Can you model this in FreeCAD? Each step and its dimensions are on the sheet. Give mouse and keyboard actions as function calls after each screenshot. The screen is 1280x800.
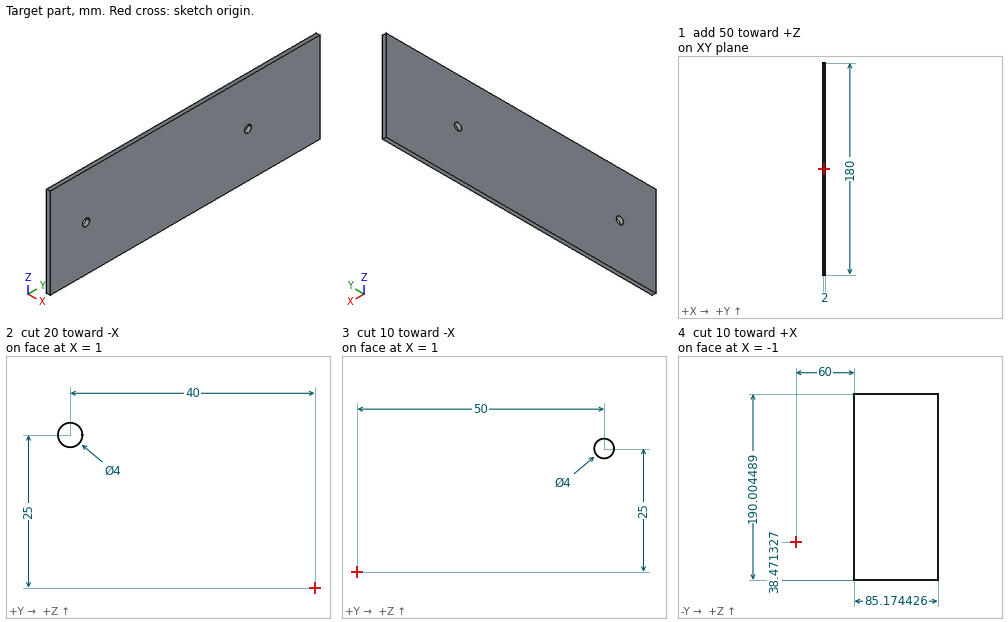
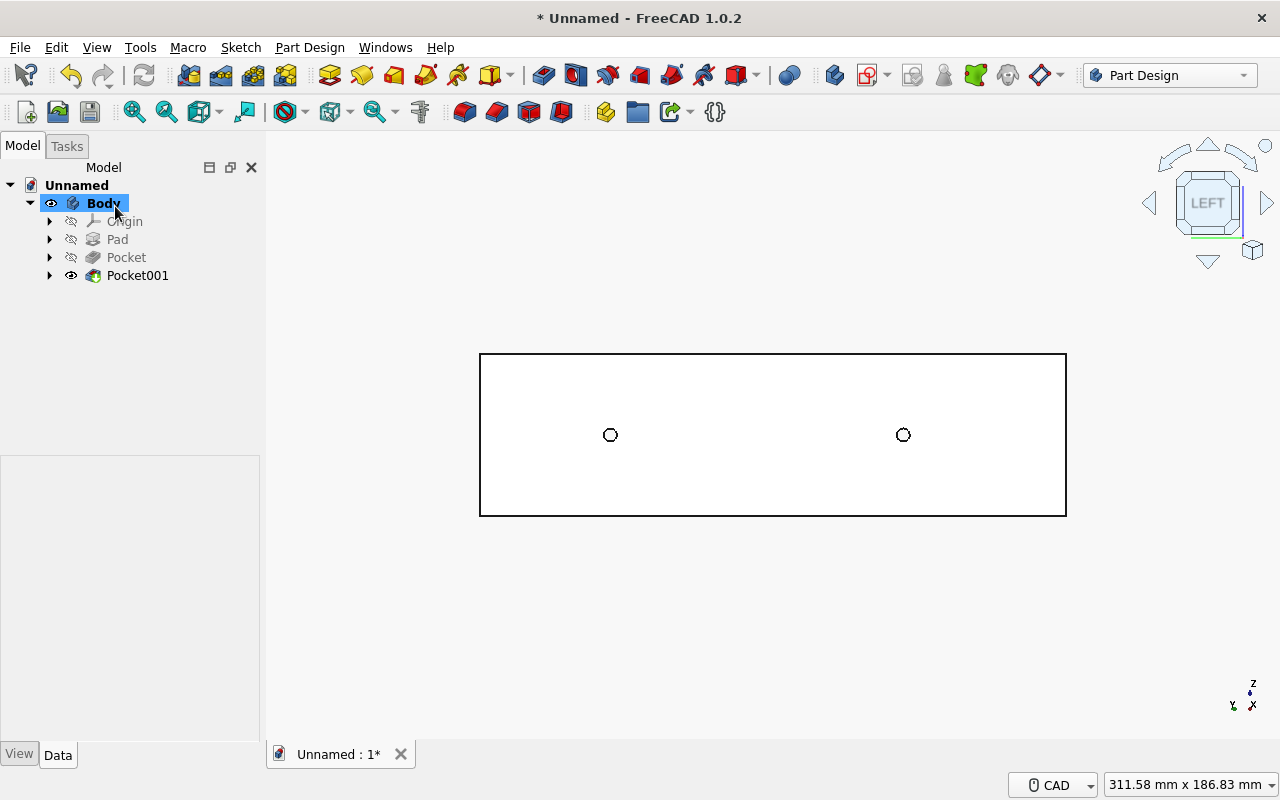
click(773, 434)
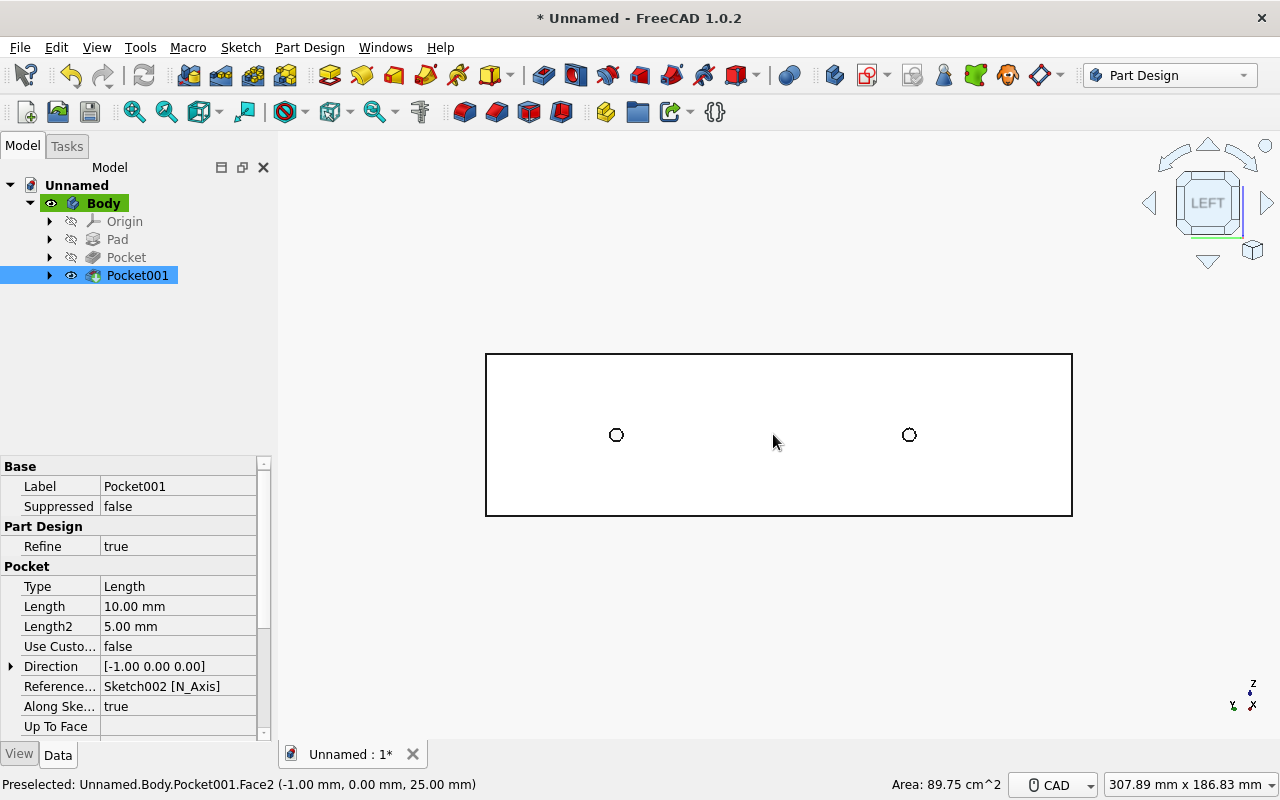
click(868, 76)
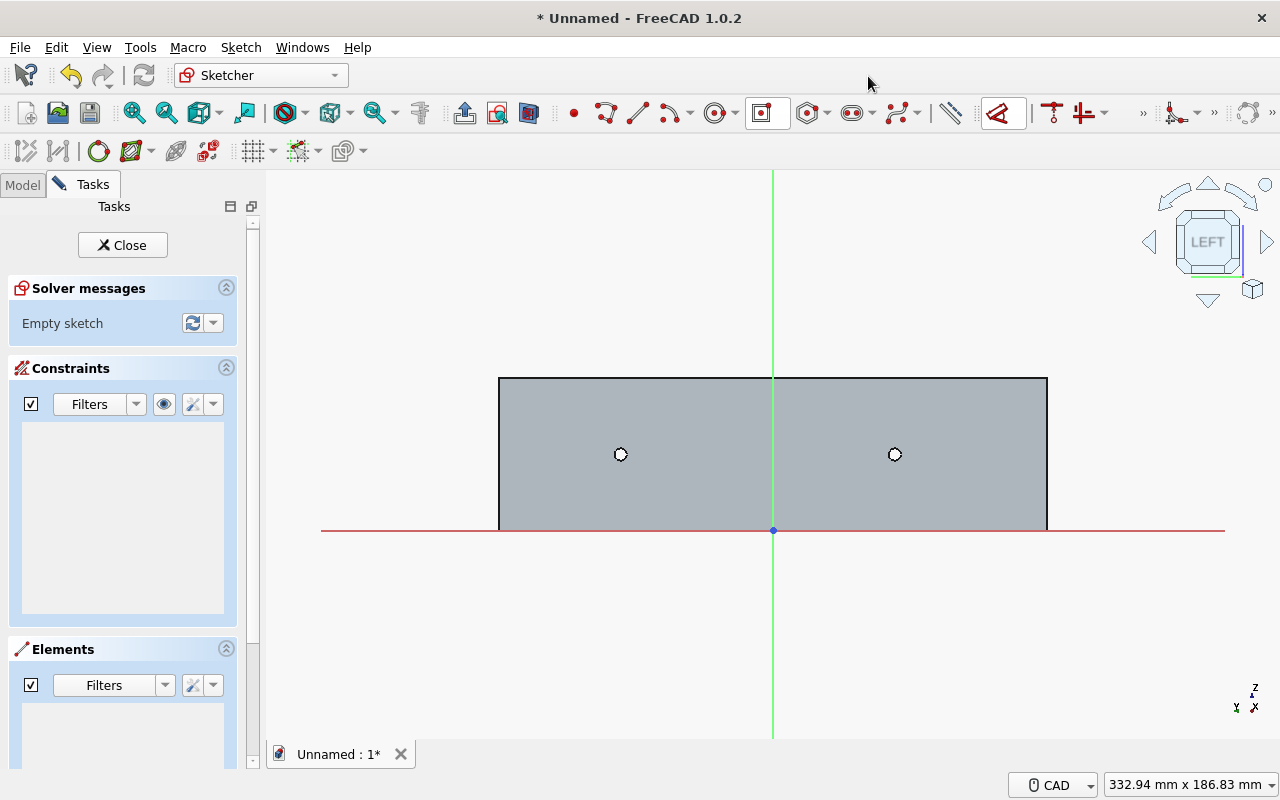
scroll(294, 650, down, 2)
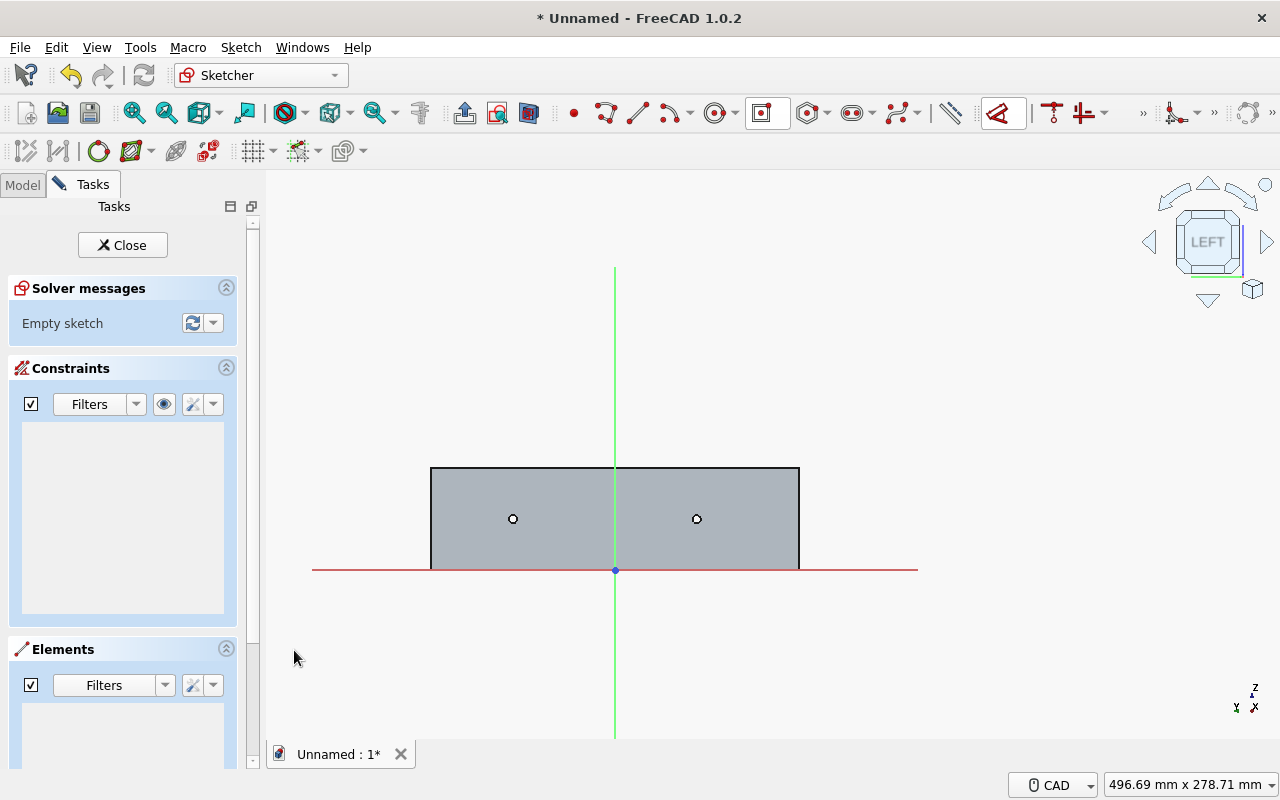
key(g)
key(r)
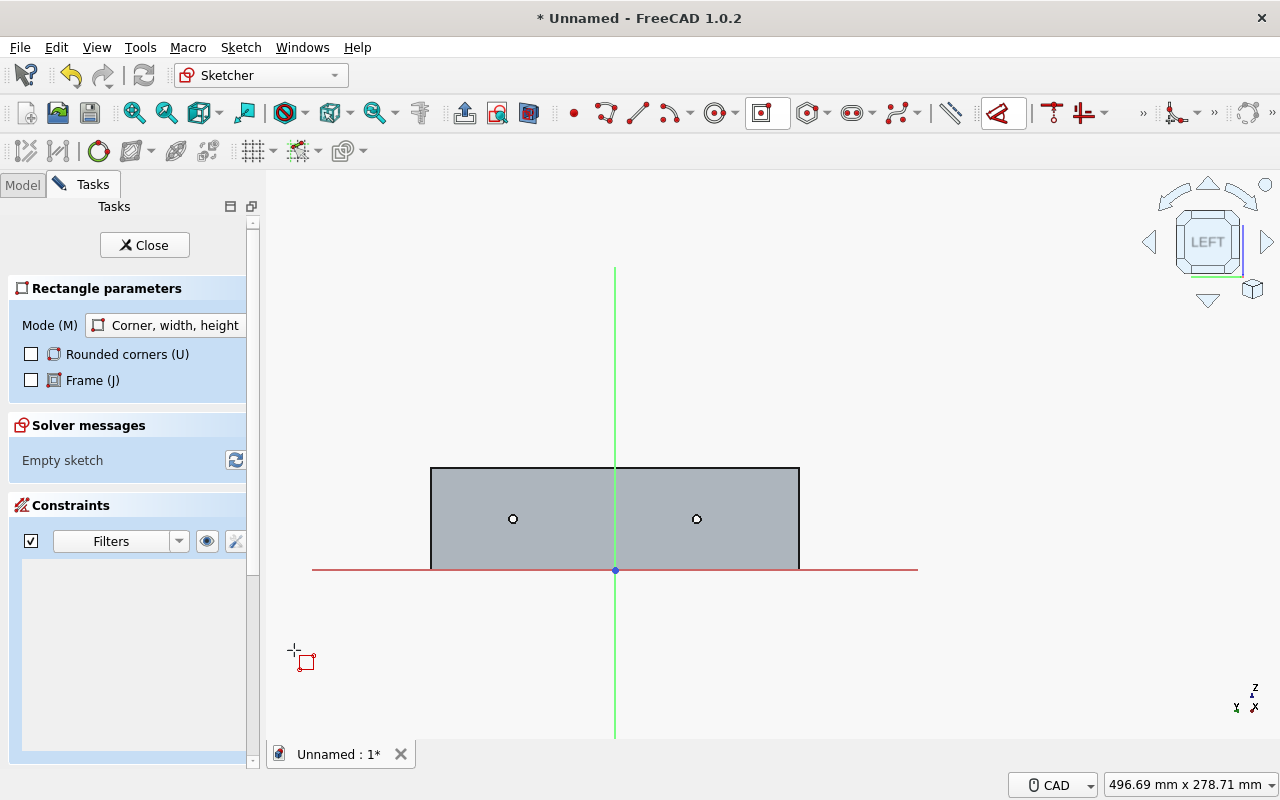
click(738, 261)
click(911, 649)
key(Escape)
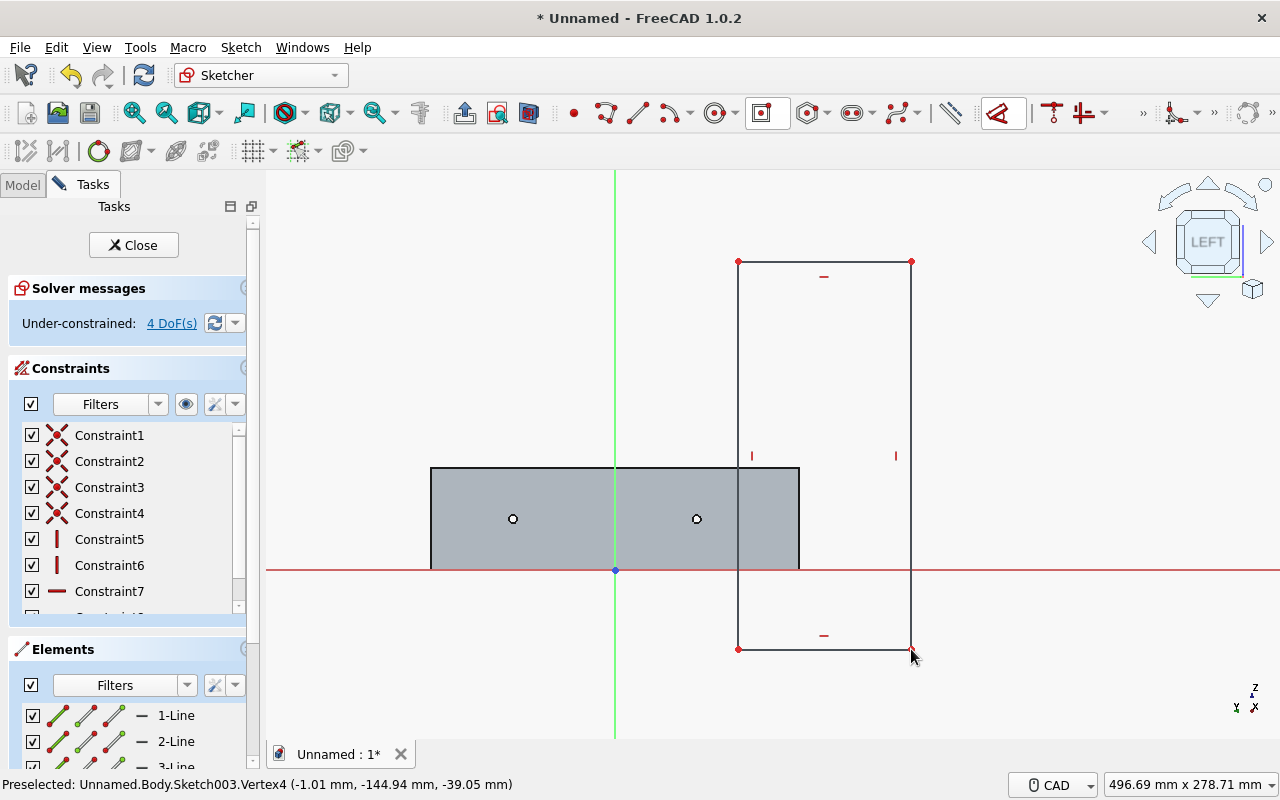
click(738, 262)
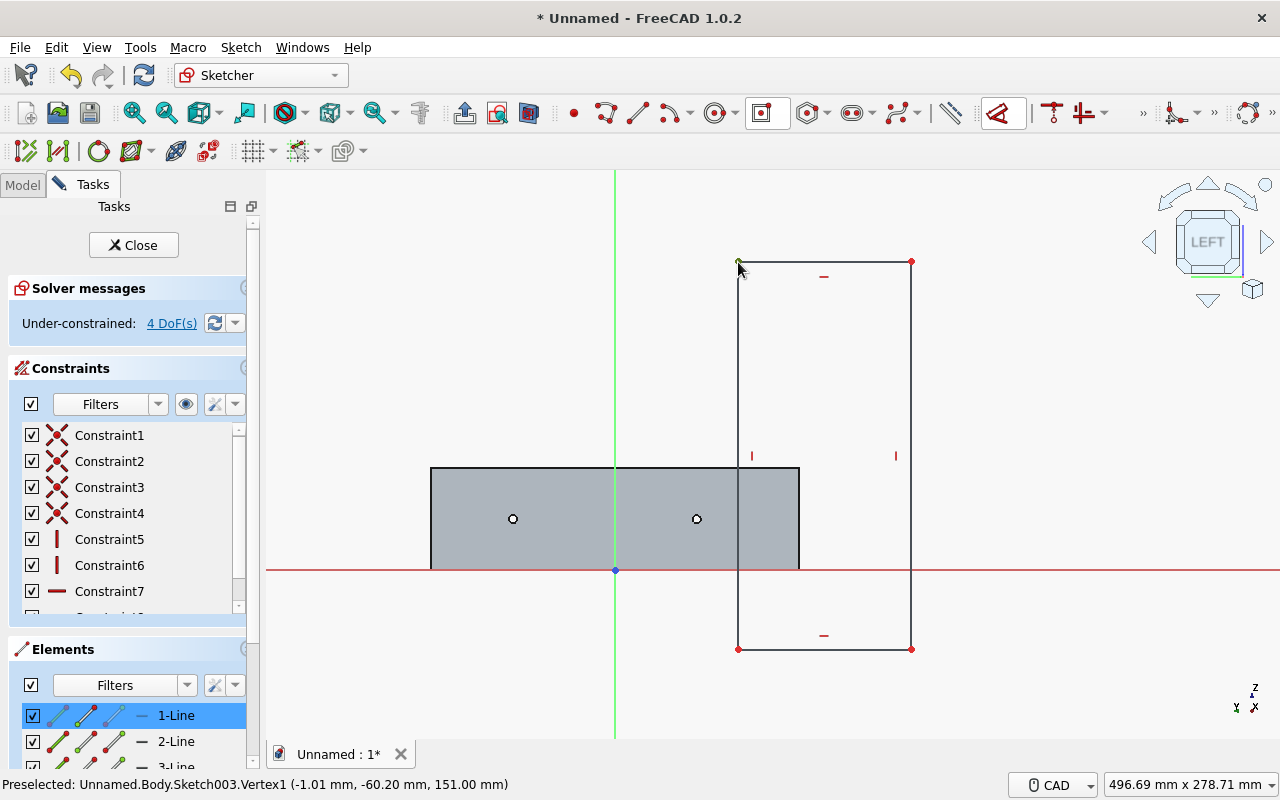
click(1020, 114)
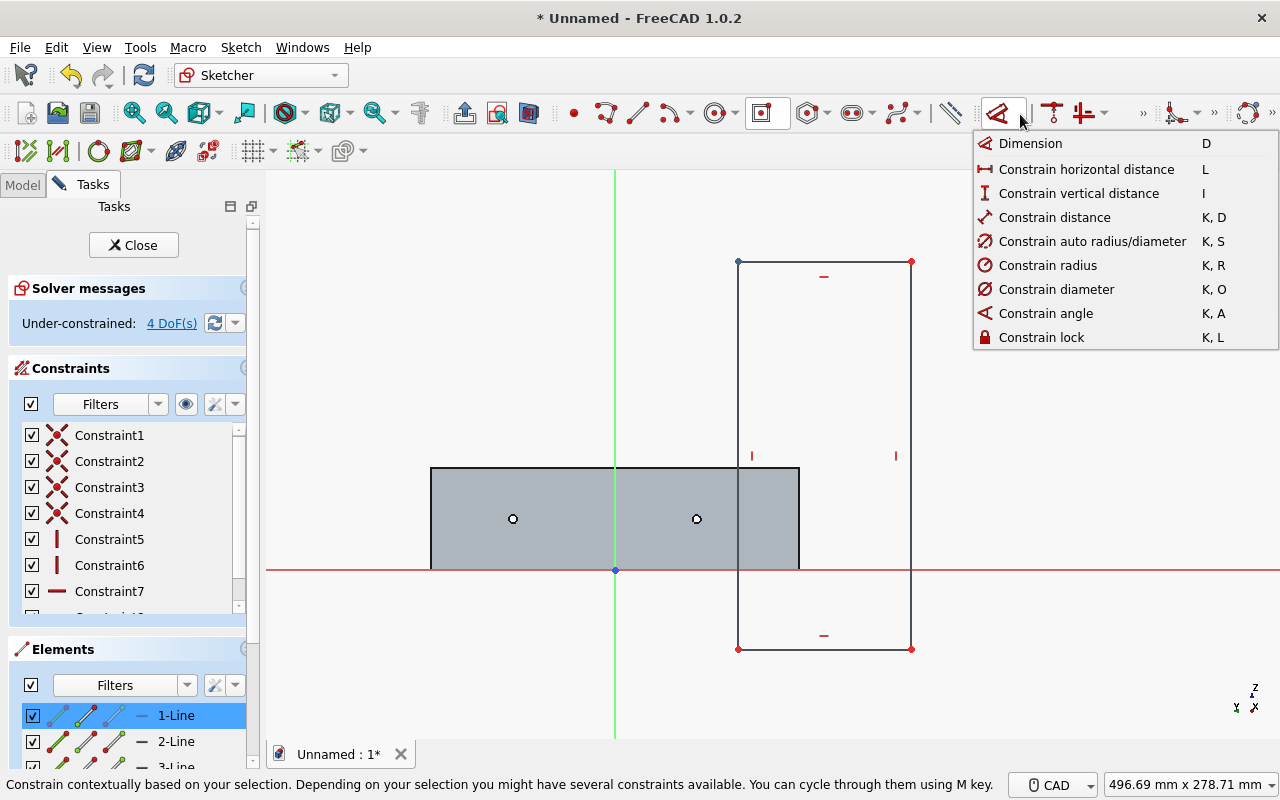
click(1126, 169)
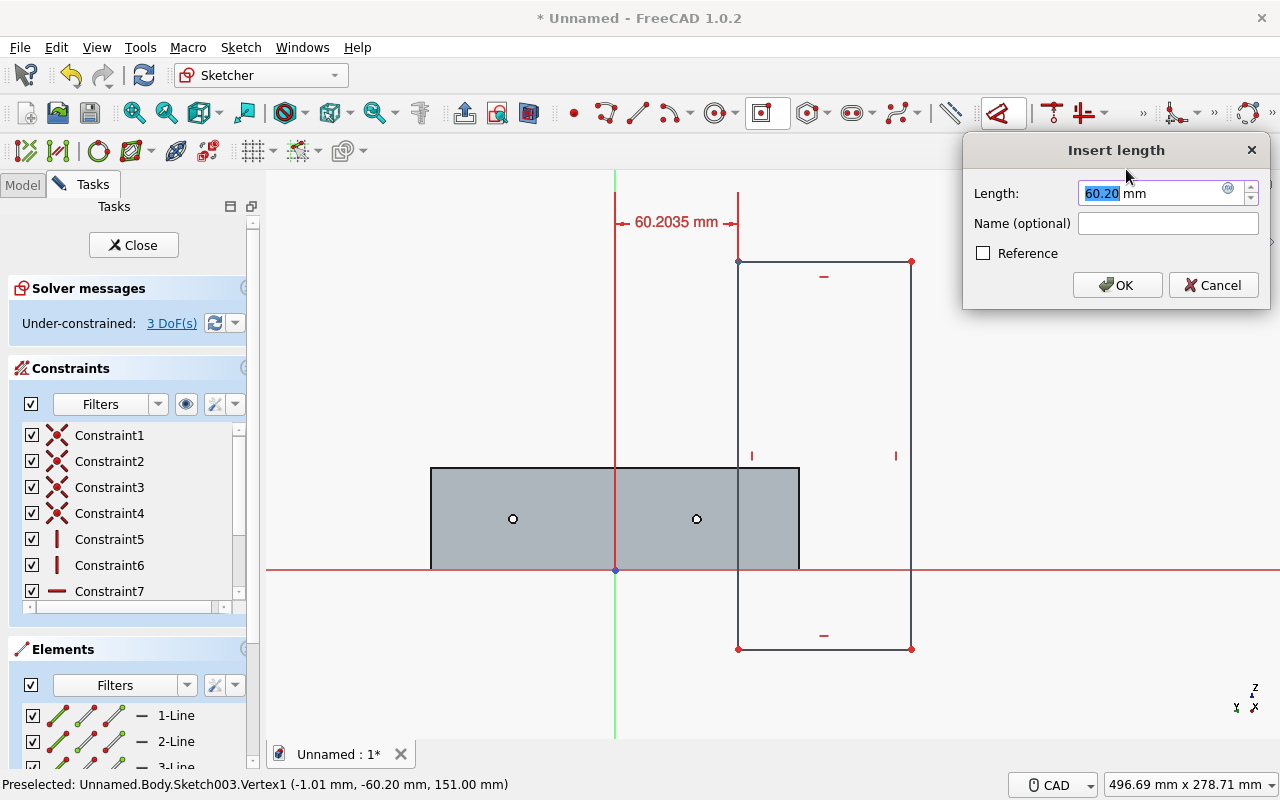
text(60)
key(Return)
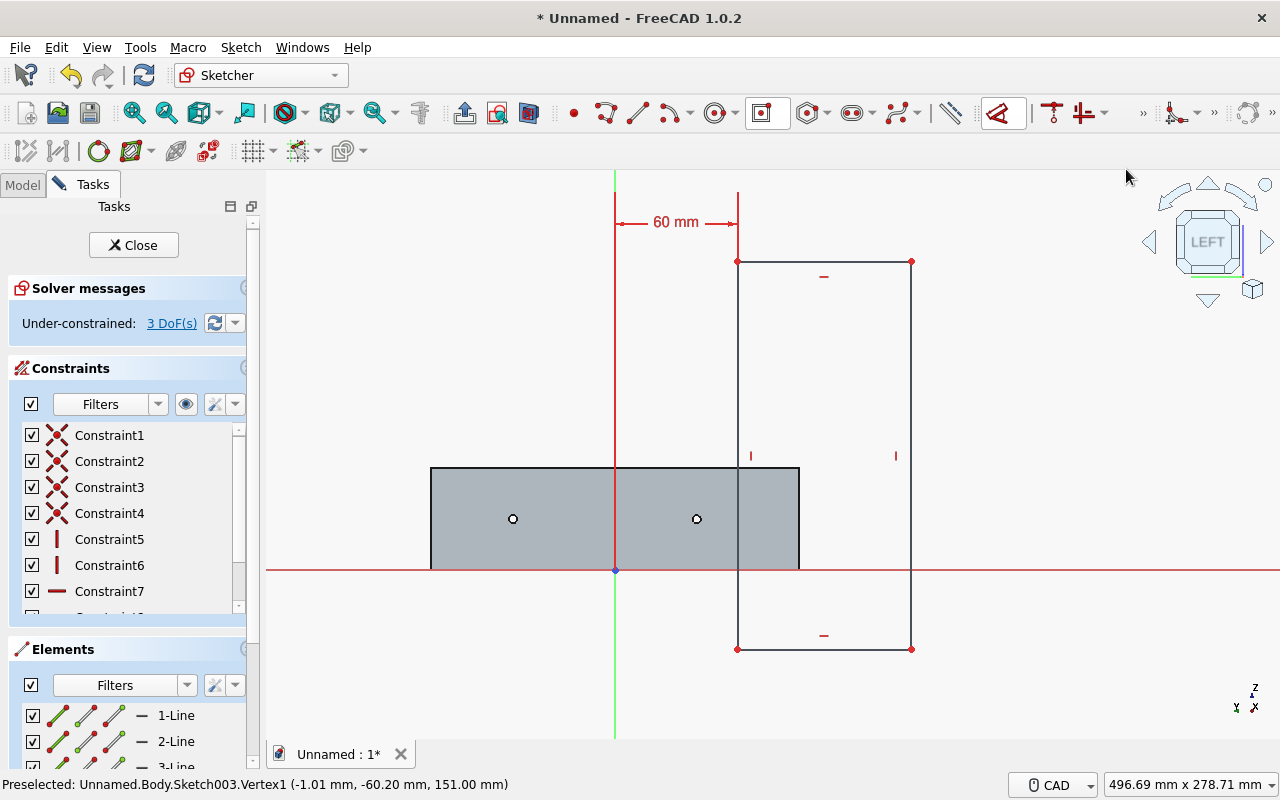
click(790, 650)